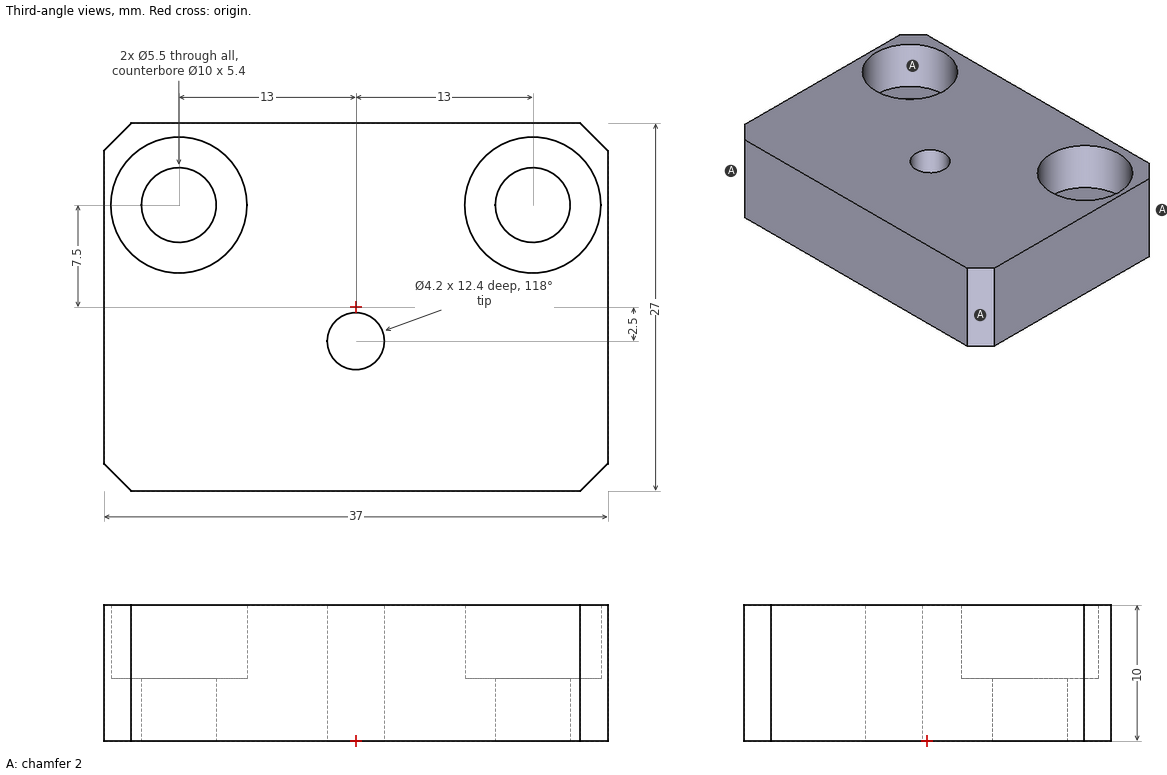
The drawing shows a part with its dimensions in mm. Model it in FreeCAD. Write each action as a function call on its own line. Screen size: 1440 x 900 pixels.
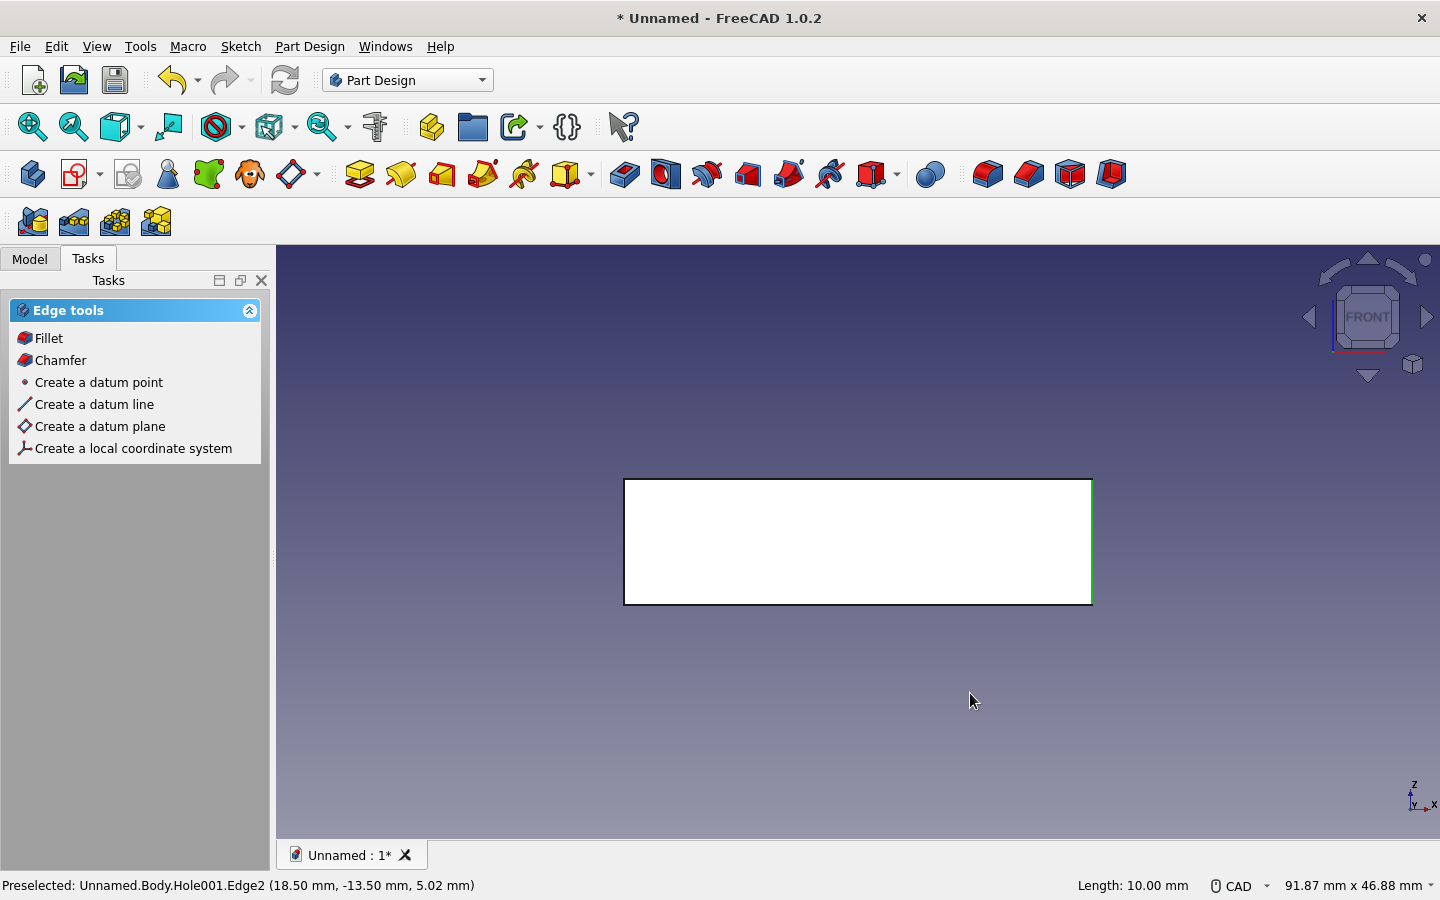
click(33, 128)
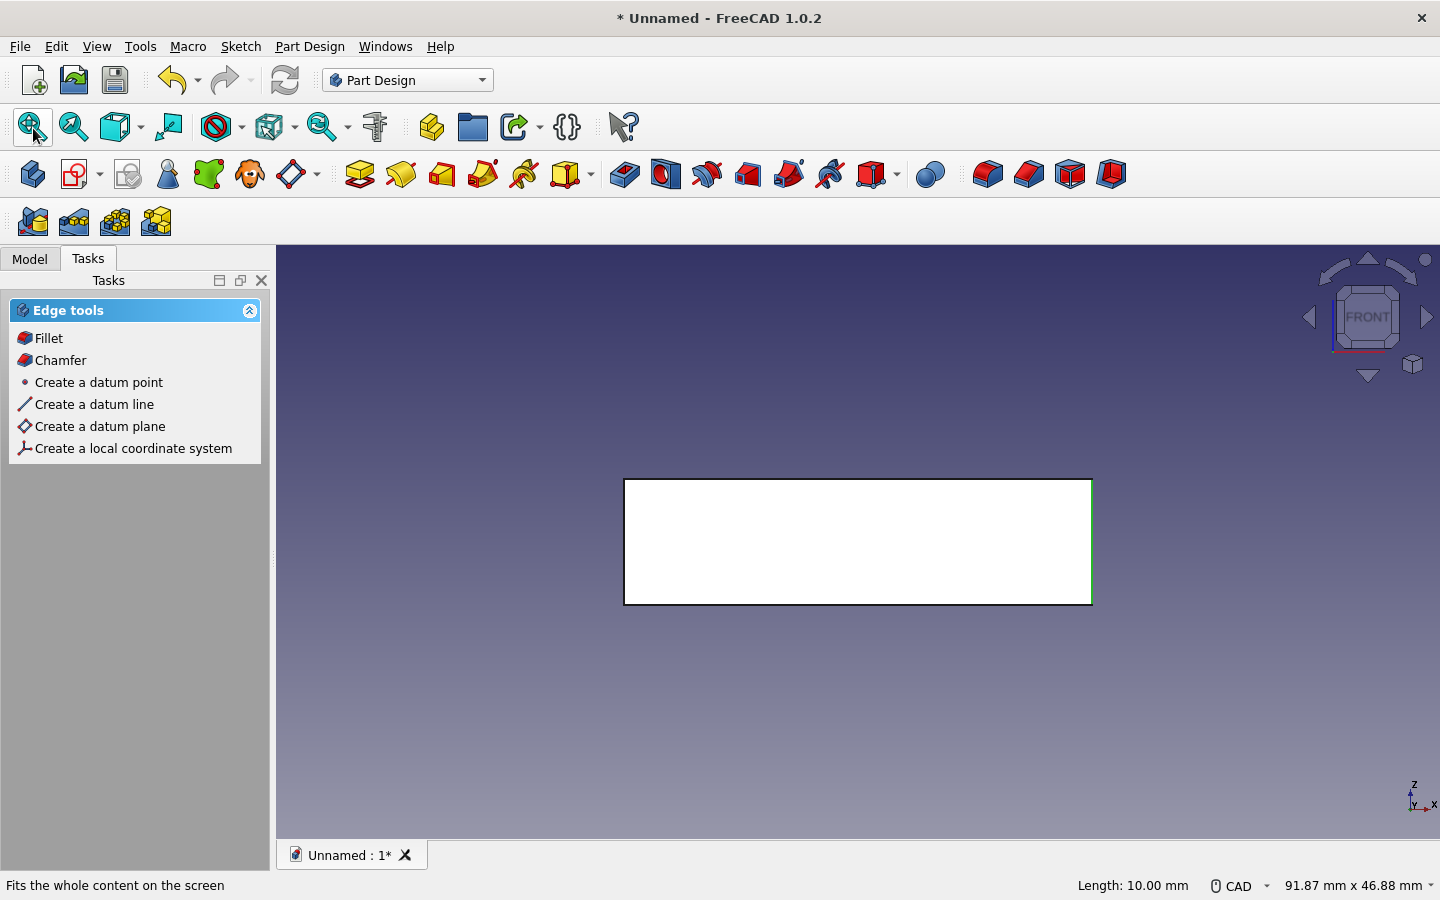
click(624, 541, ctrl)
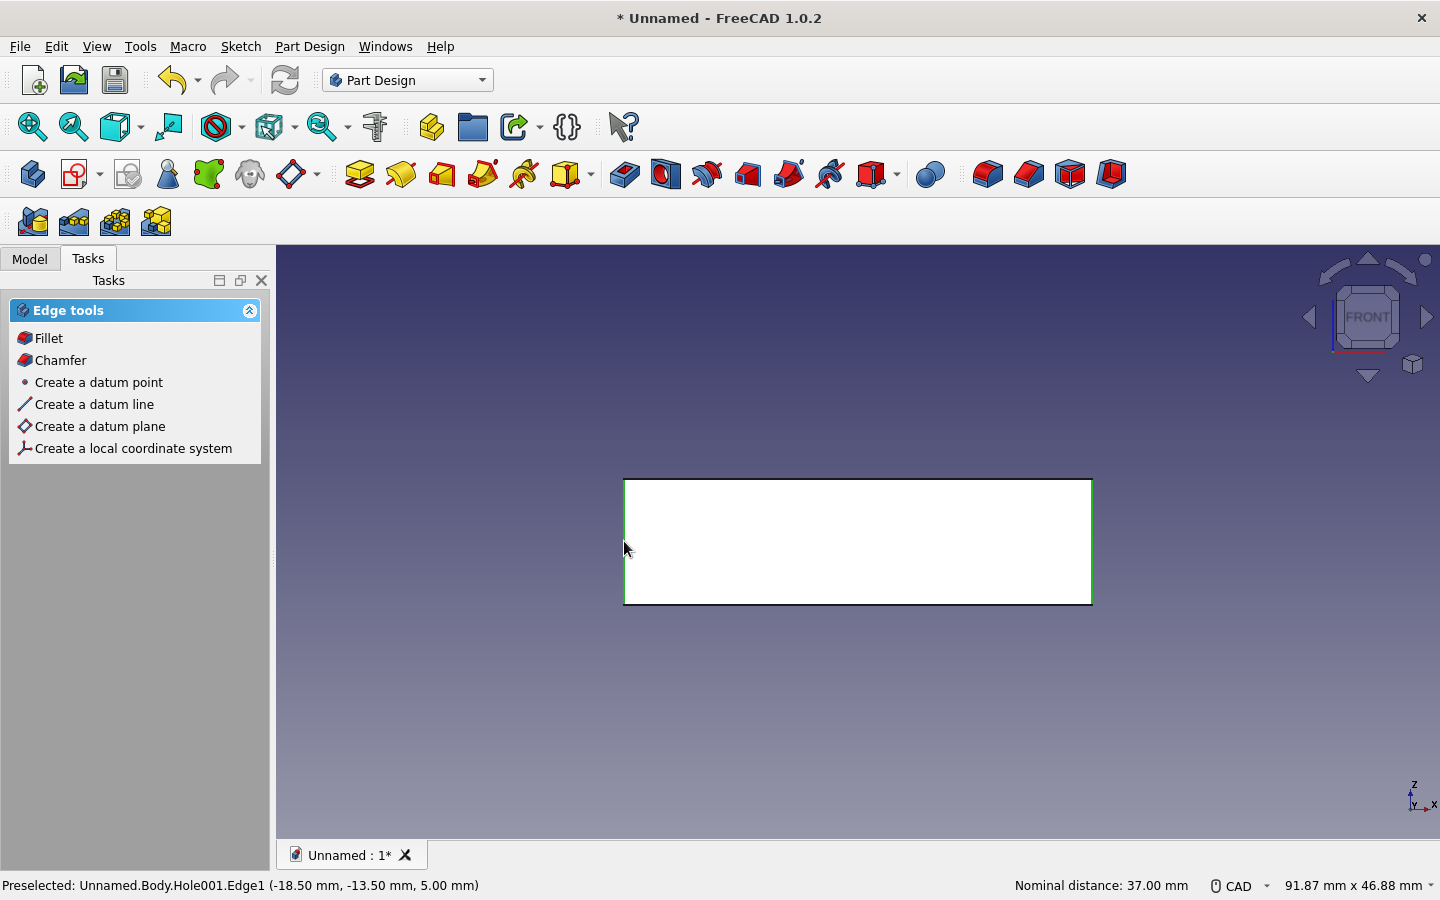
key(3)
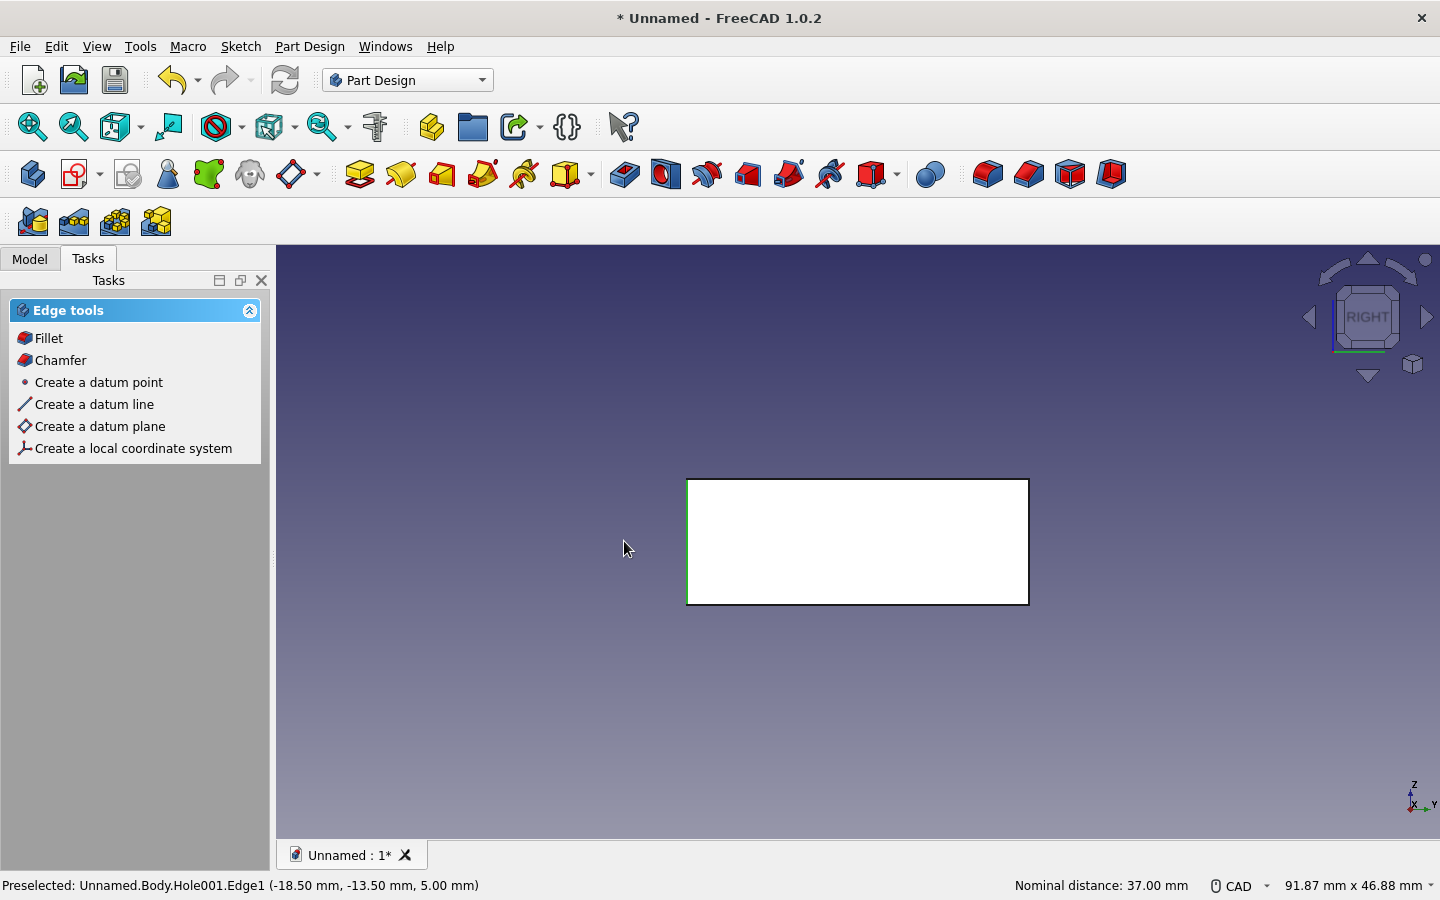
click(33, 128)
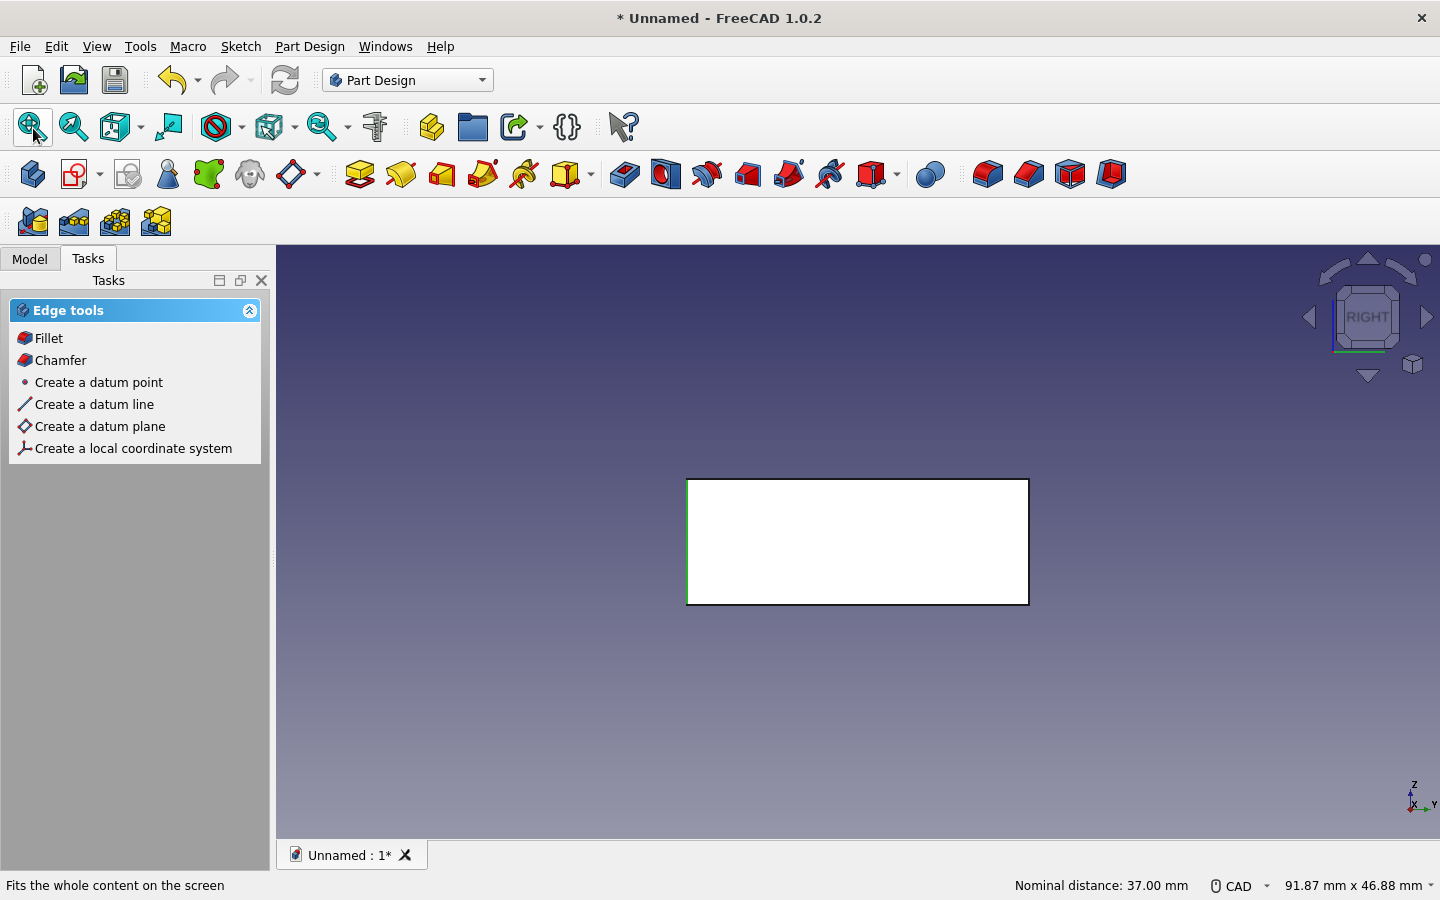
click(1029, 541, ctrl)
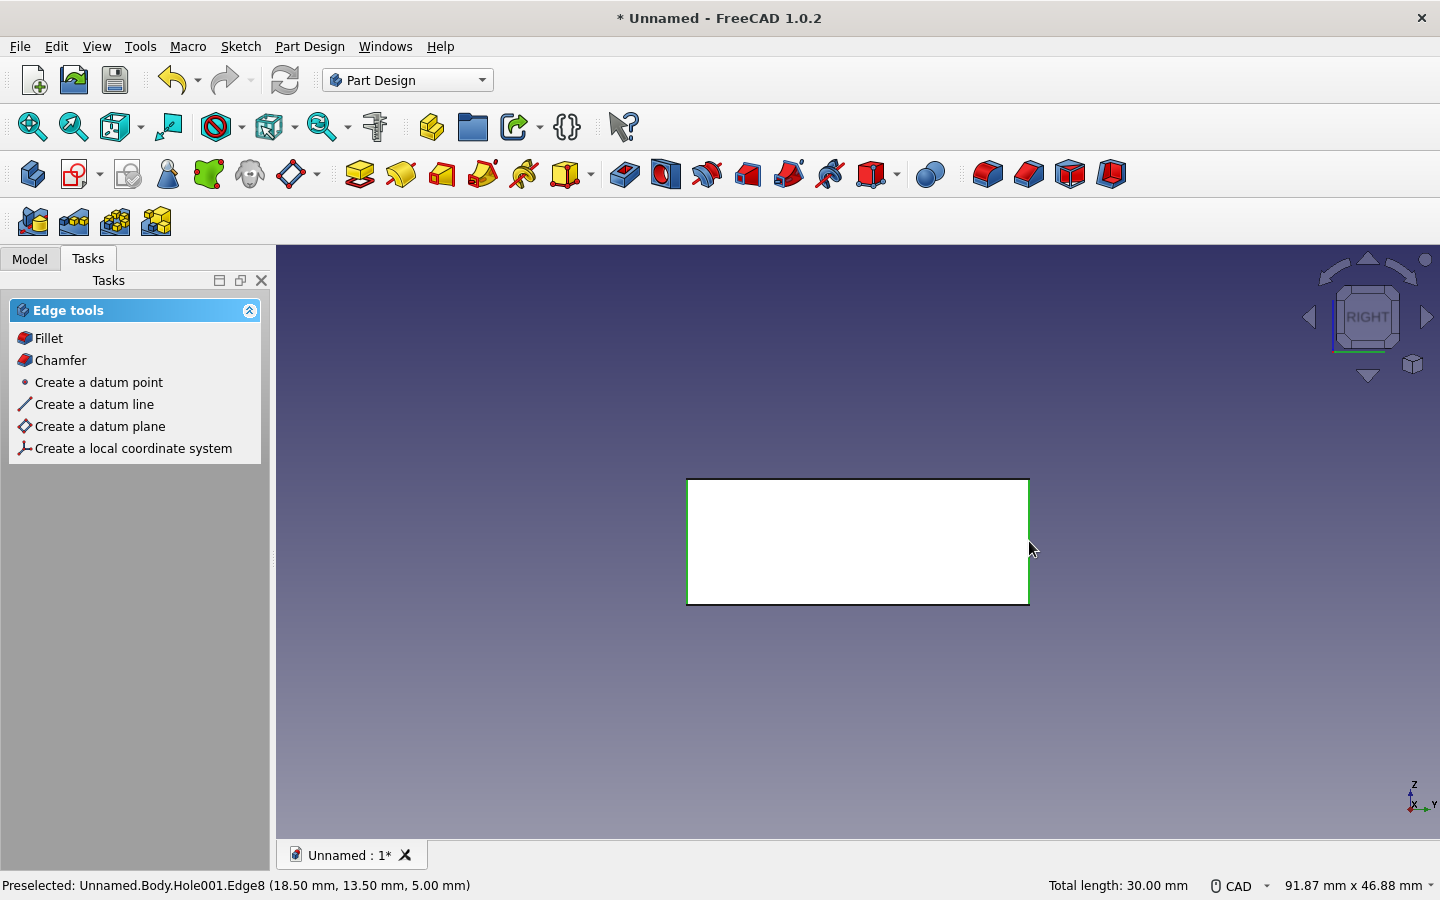
key(5)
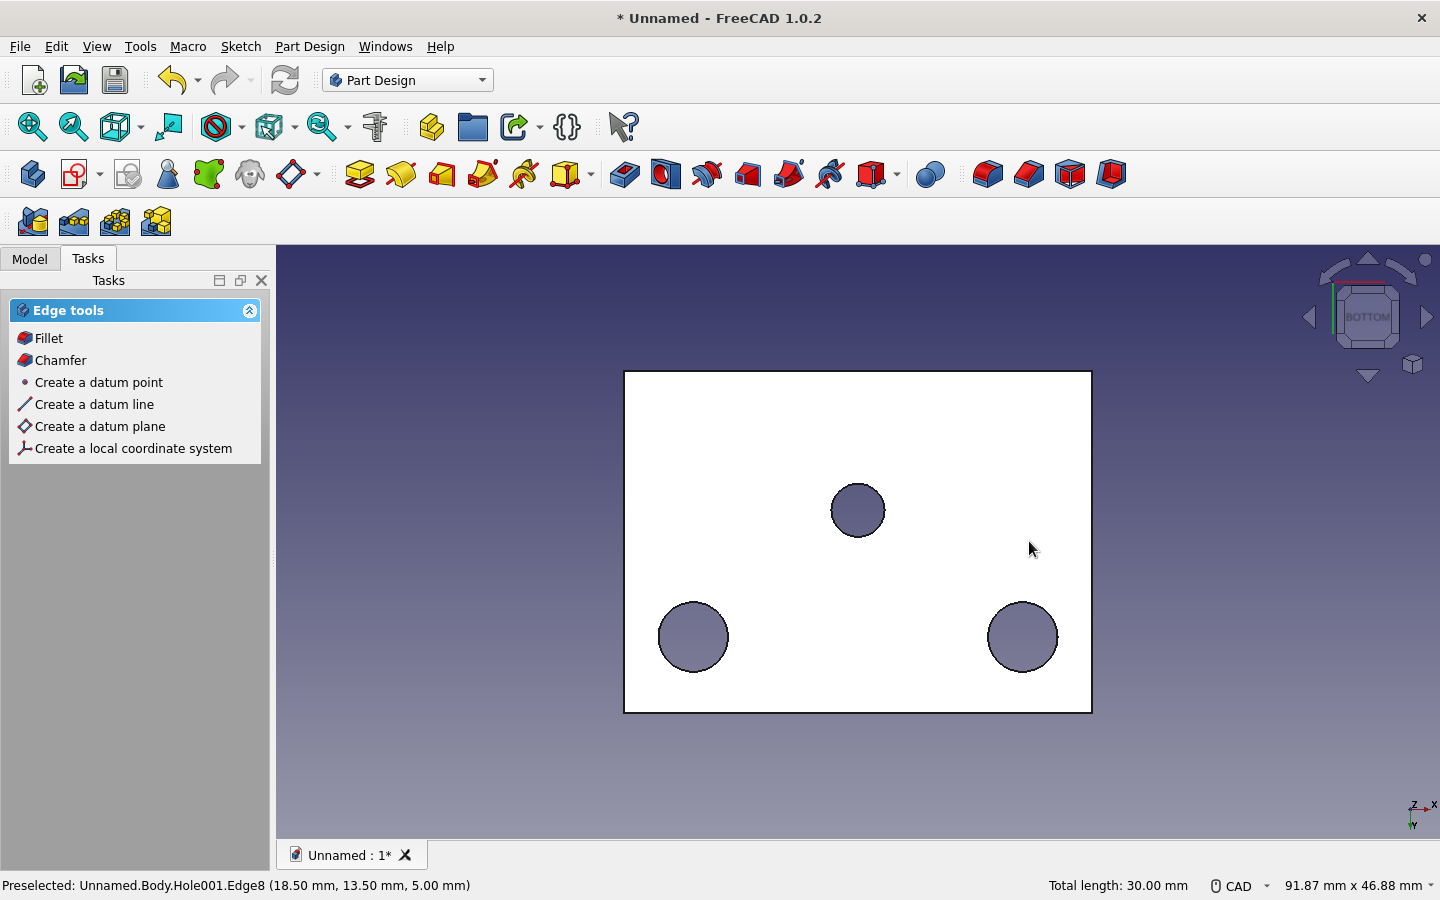
key(4)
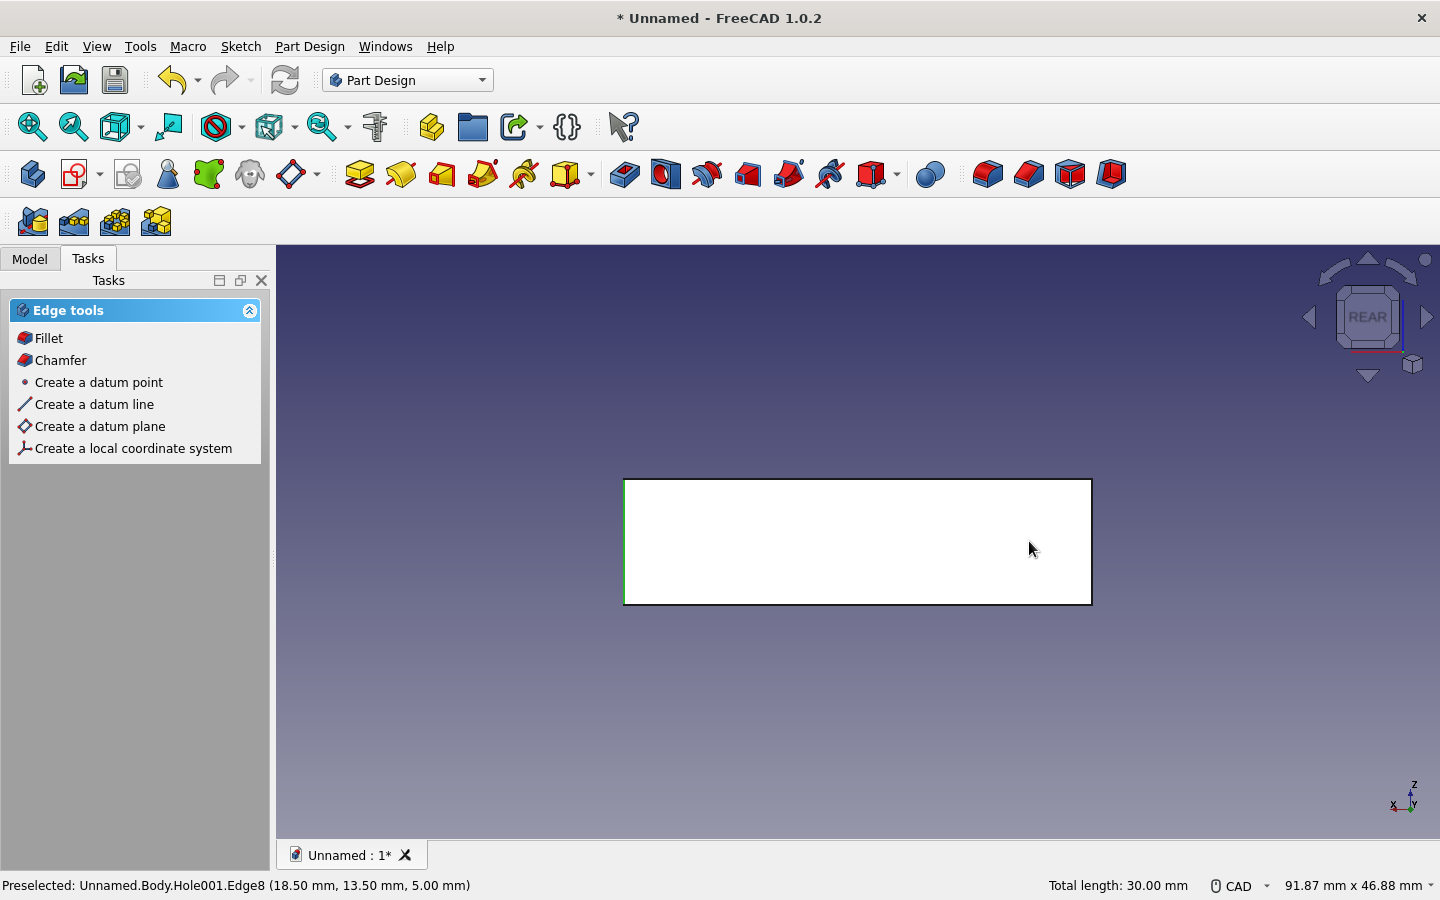
click(33, 128)